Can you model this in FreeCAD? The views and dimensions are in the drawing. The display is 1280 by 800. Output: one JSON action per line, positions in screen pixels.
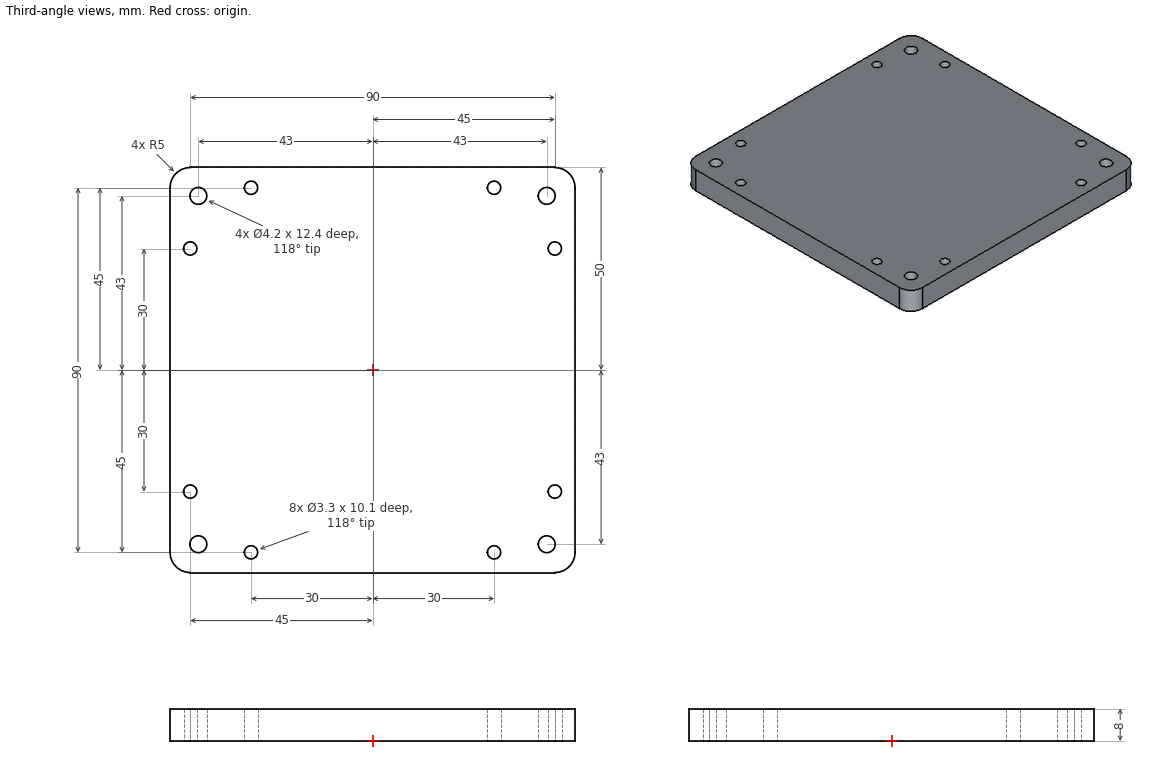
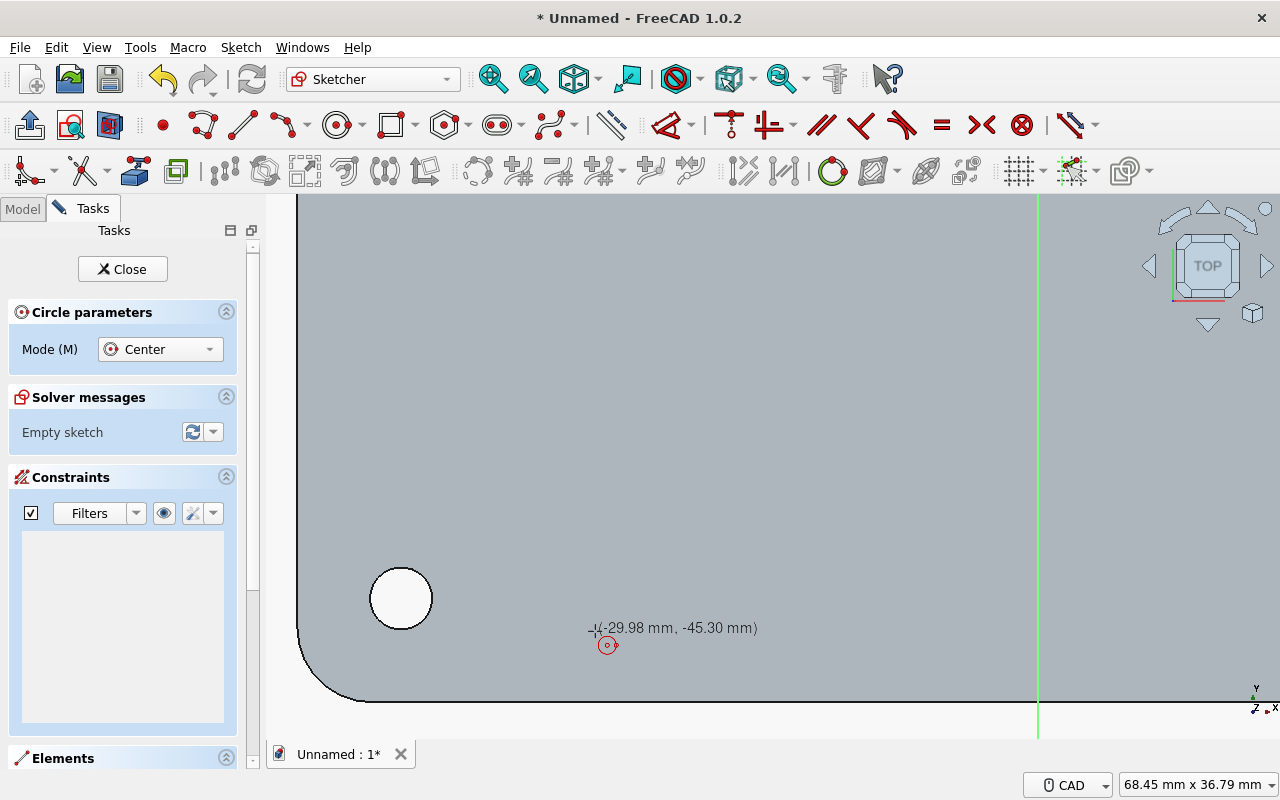
{"action": "scroll", "coordinate": [595, 632], "scroll_direction": "down", "scroll_amount": 7}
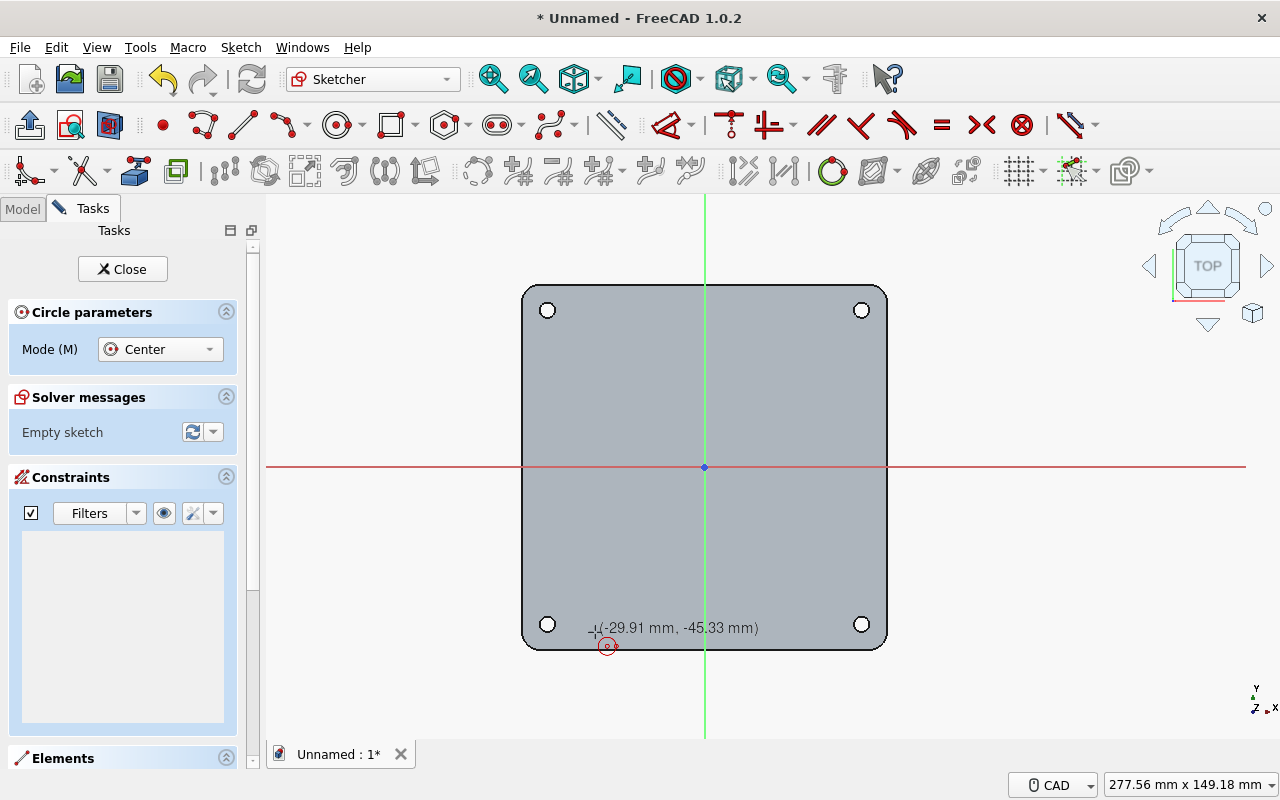
{"action": "left_click", "coordinate": [595, 632]}
{"action": "mouse_move", "coordinate": [599, 627]}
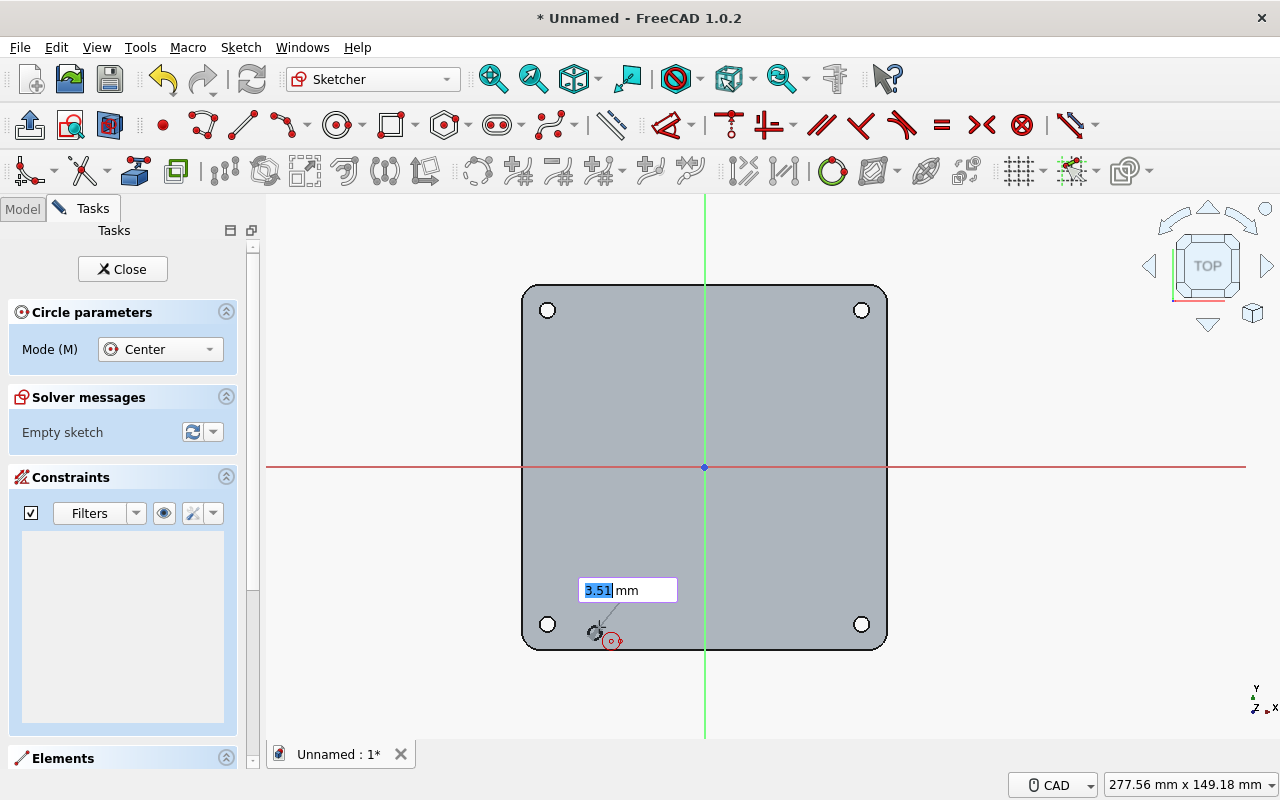
{"action": "type", "text": "3.3"}
{"action": "key", "text": "Return"}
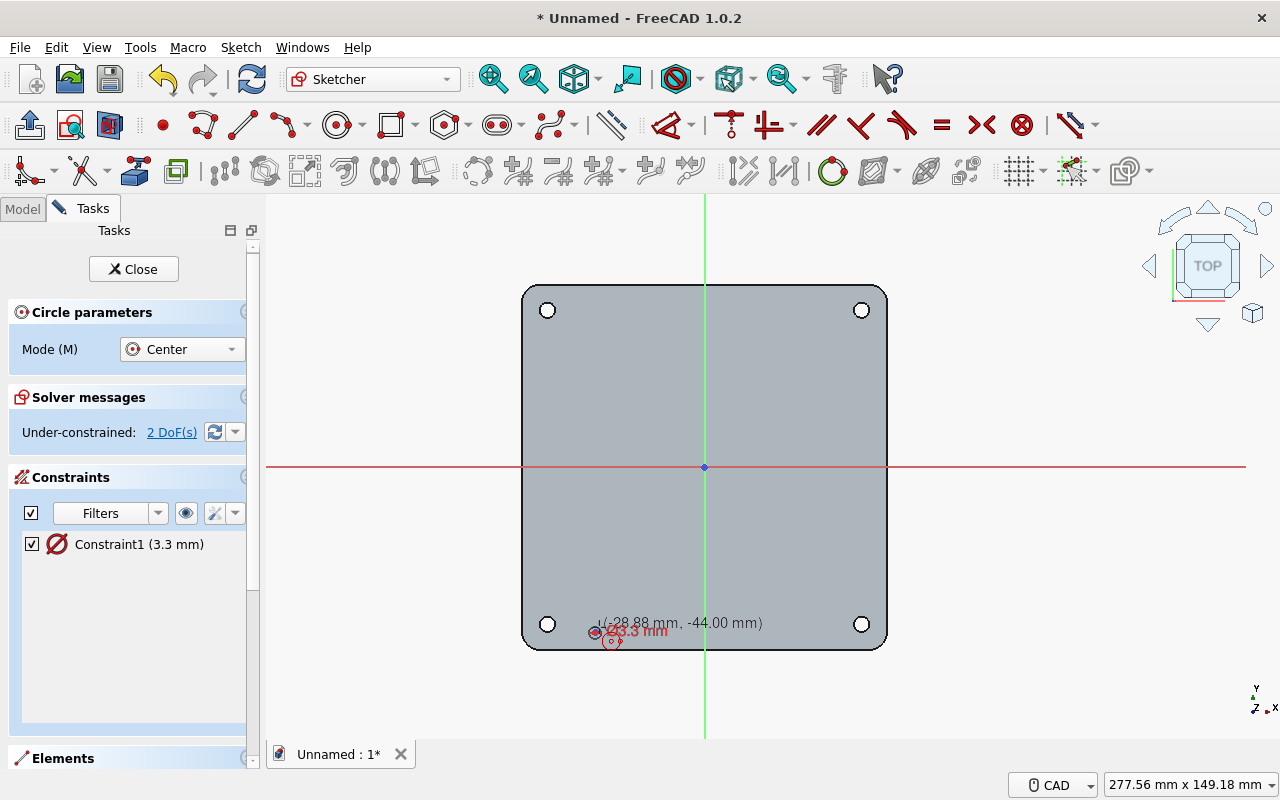
{"action": "scroll", "coordinate": [814, 632], "scroll_direction": "up", "scroll_amount": 7}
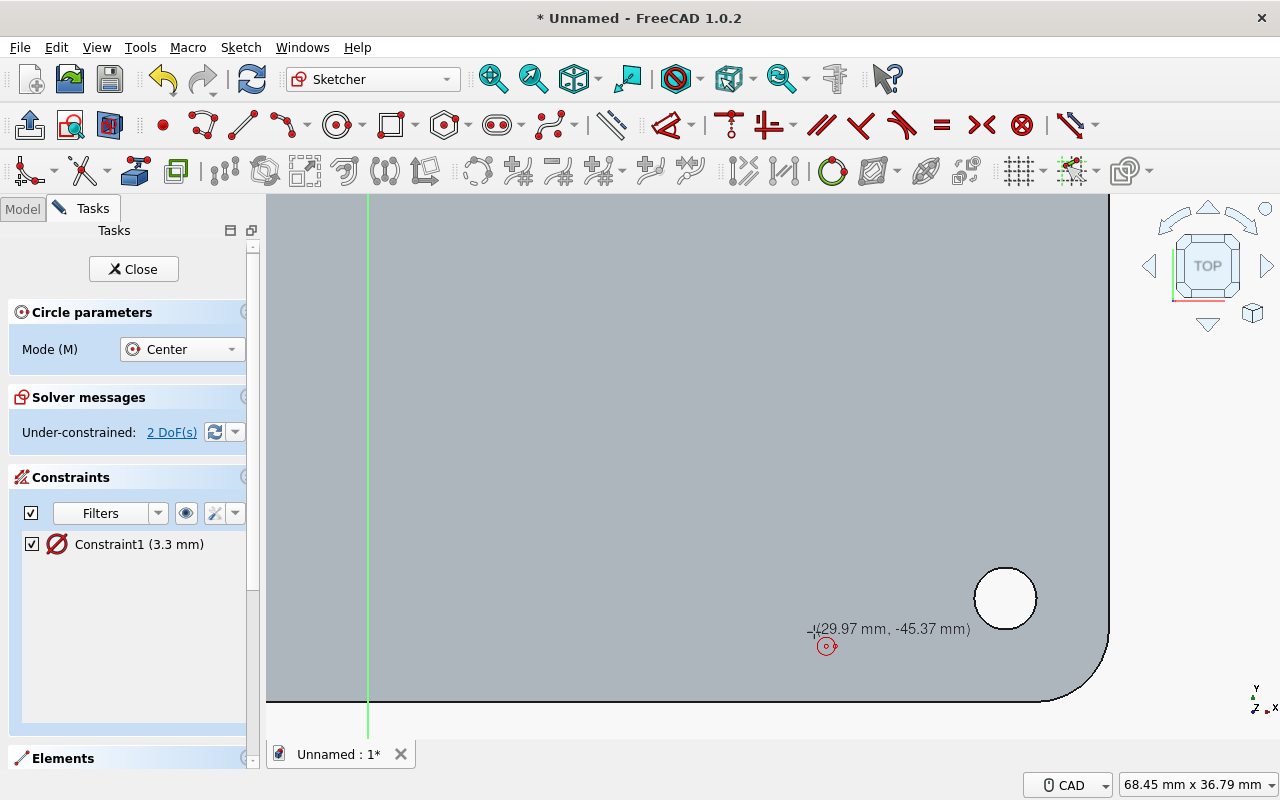
{"action": "scroll", "coordinate": [815, 632], "scroll_direction": "down", "scroll_amount": 7}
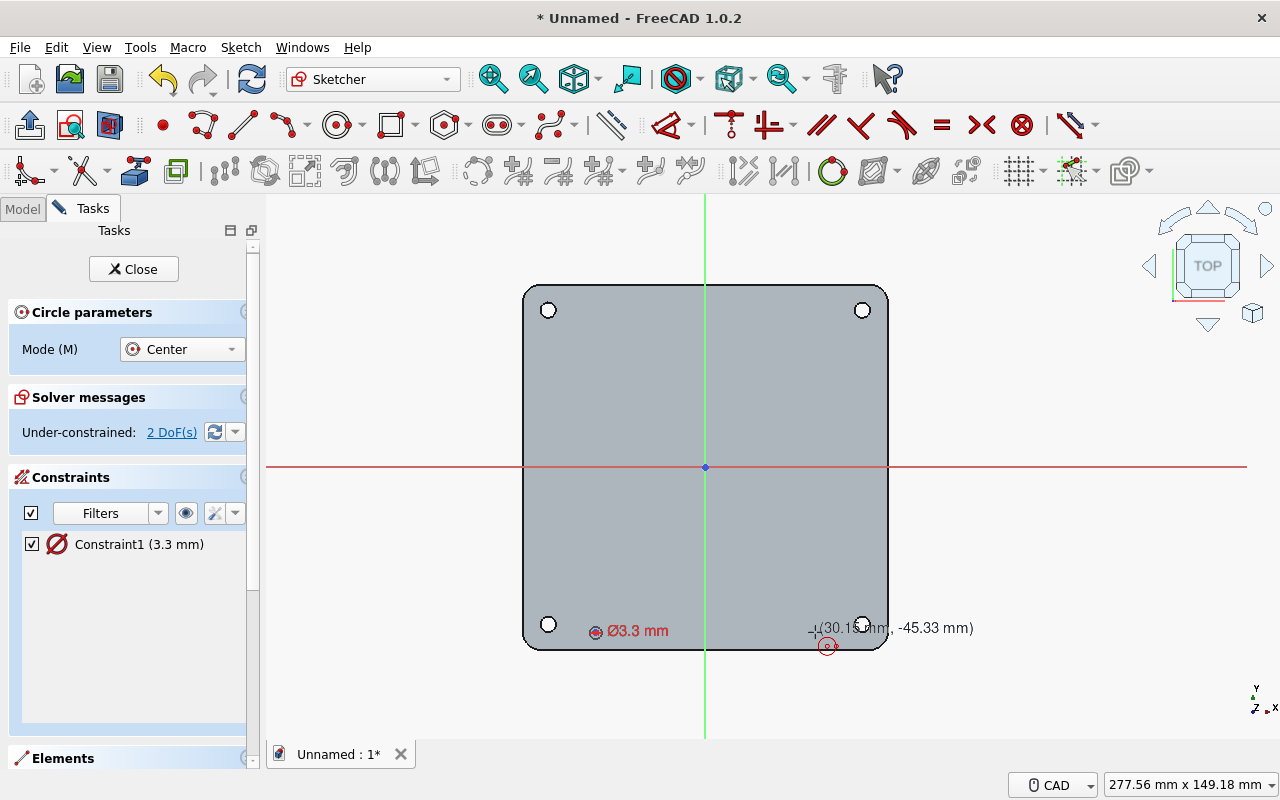
{"action": "left_click", "coordinate": [815, 632]}
{"action": "mouse_move", "coordinate": [819, 627]}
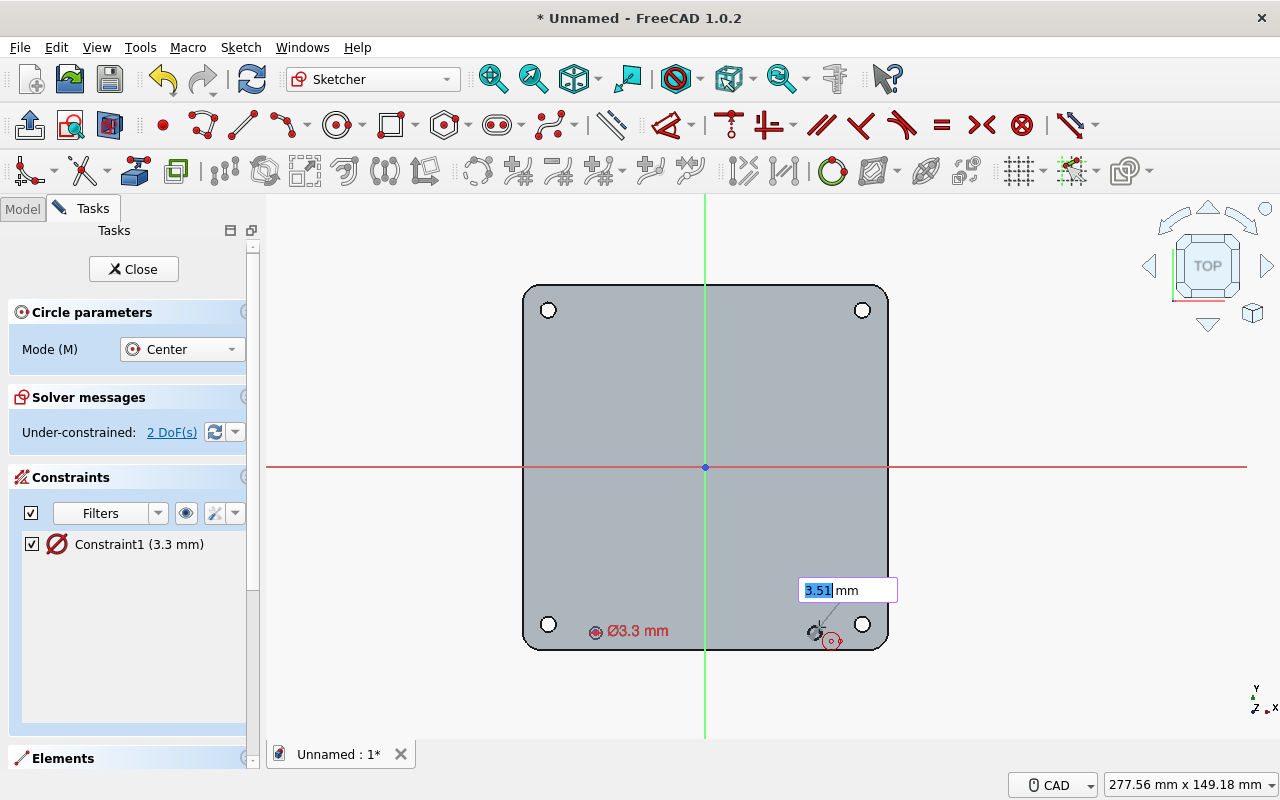
{"action": "type", "text": "3.3"}
{"action": "key", "text": "Return"}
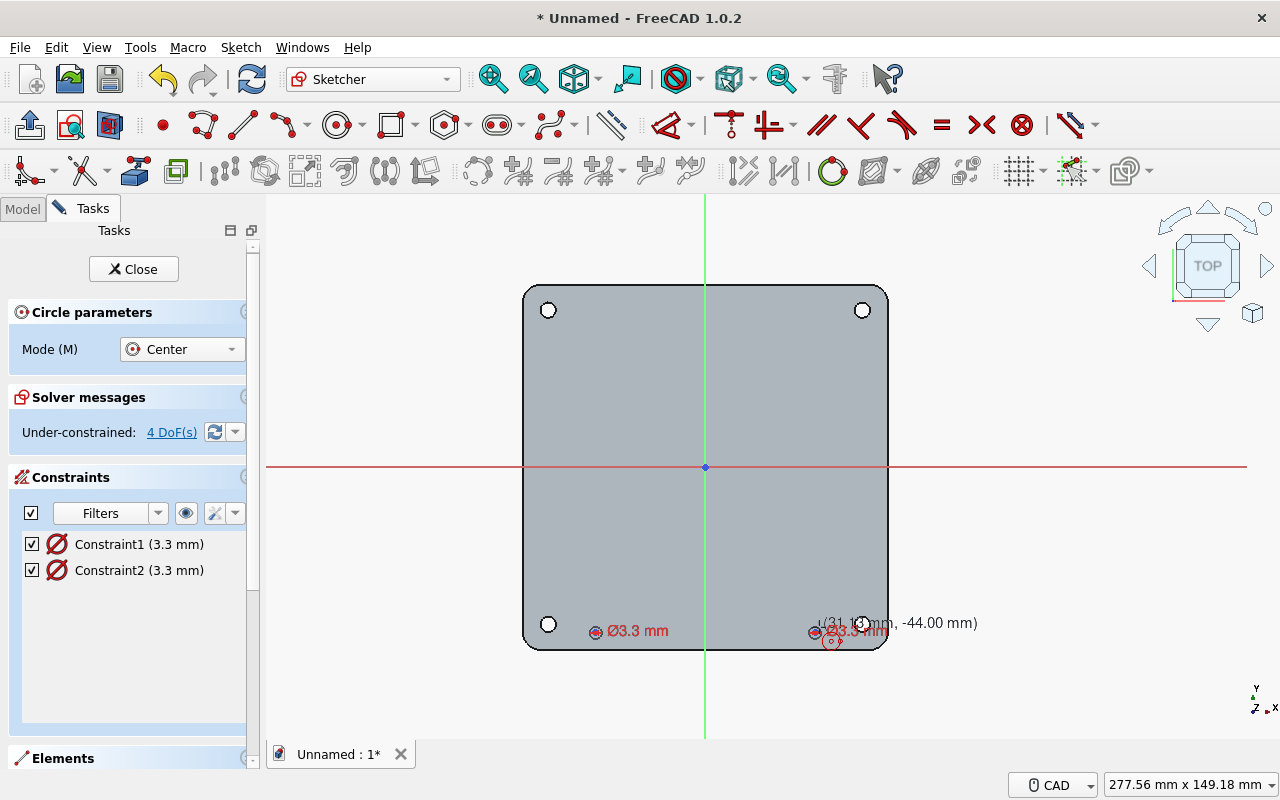
{"action": "scroll", "coordinate": [541, 577], "scroll_direction": "up", "scroll_amount": 7}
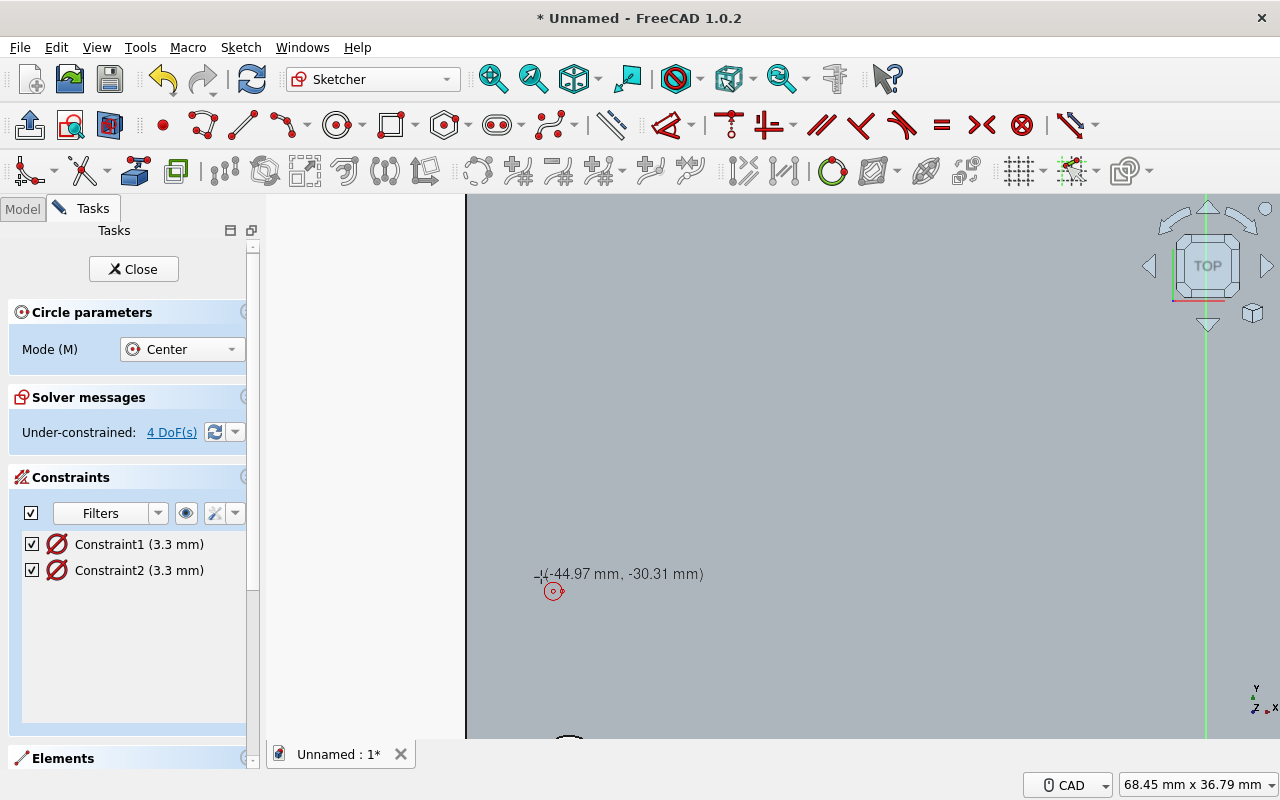
{"action": "scroll", "coordinate": [540, 577], "scroll_direction": "down", "scroll_amount": 7}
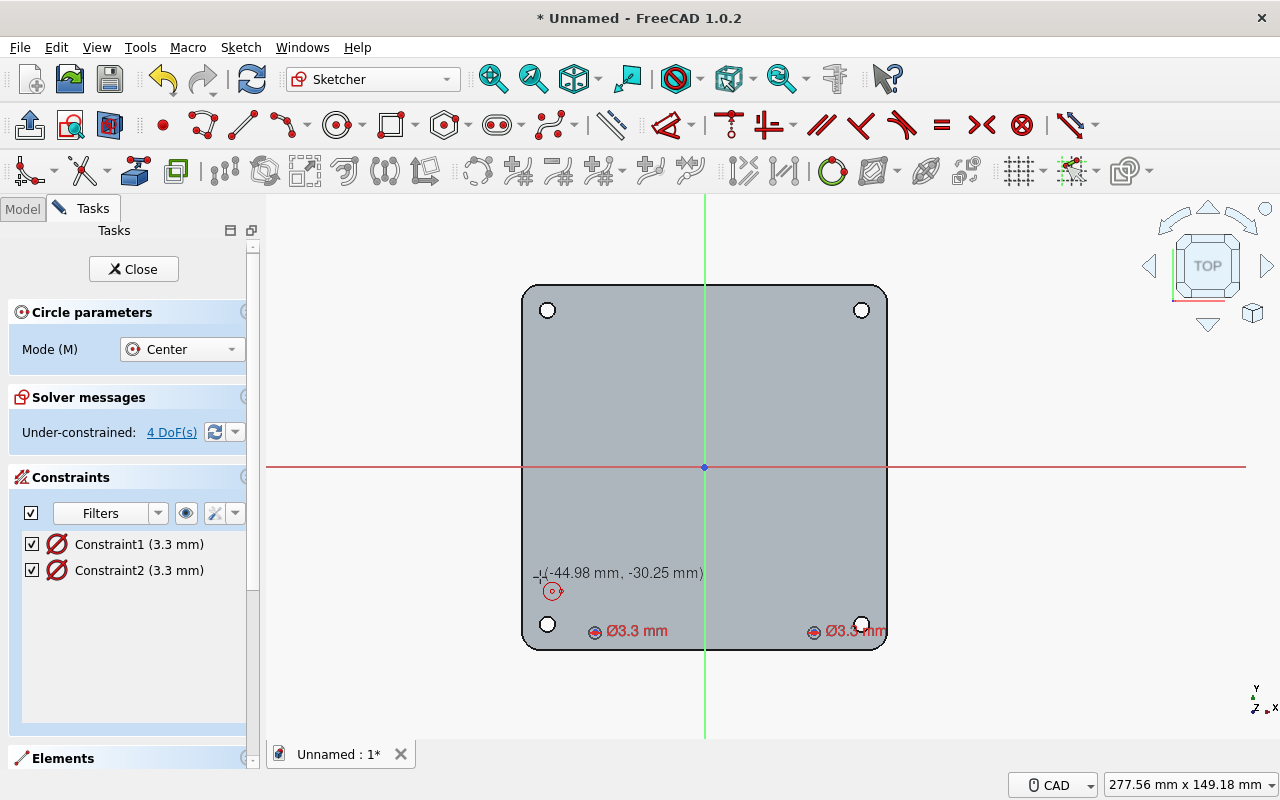
{"action": "left_click", "coordinate": [540, 577]}
{"action": "mouse_move", "coordinate": [544, 573]}